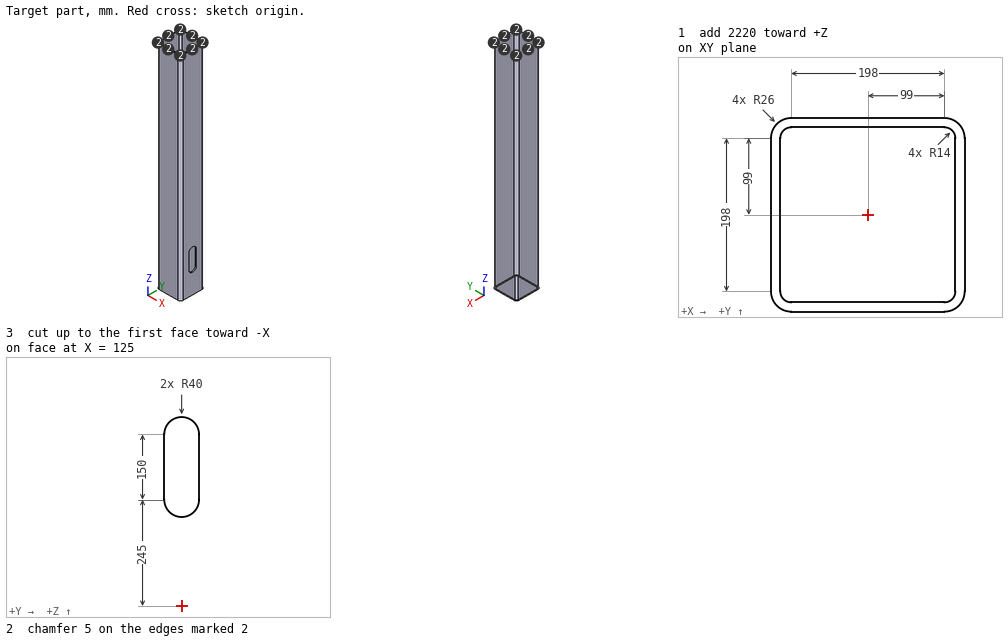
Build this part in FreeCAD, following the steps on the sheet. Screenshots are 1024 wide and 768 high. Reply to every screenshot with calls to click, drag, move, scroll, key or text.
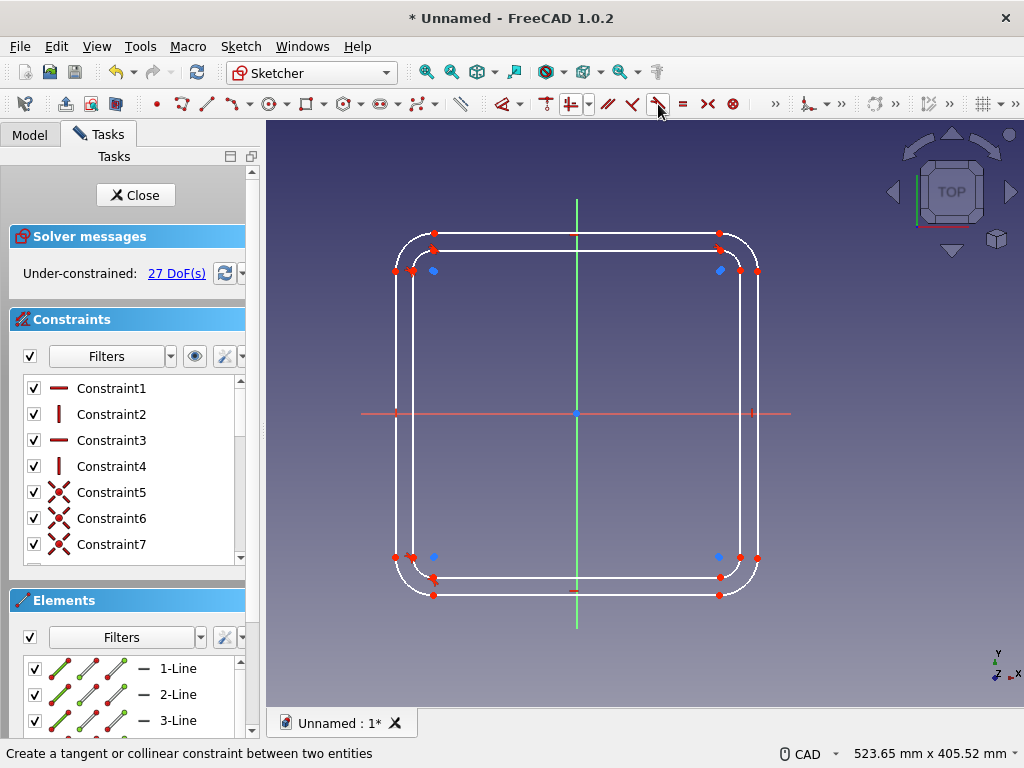
click(520, 595)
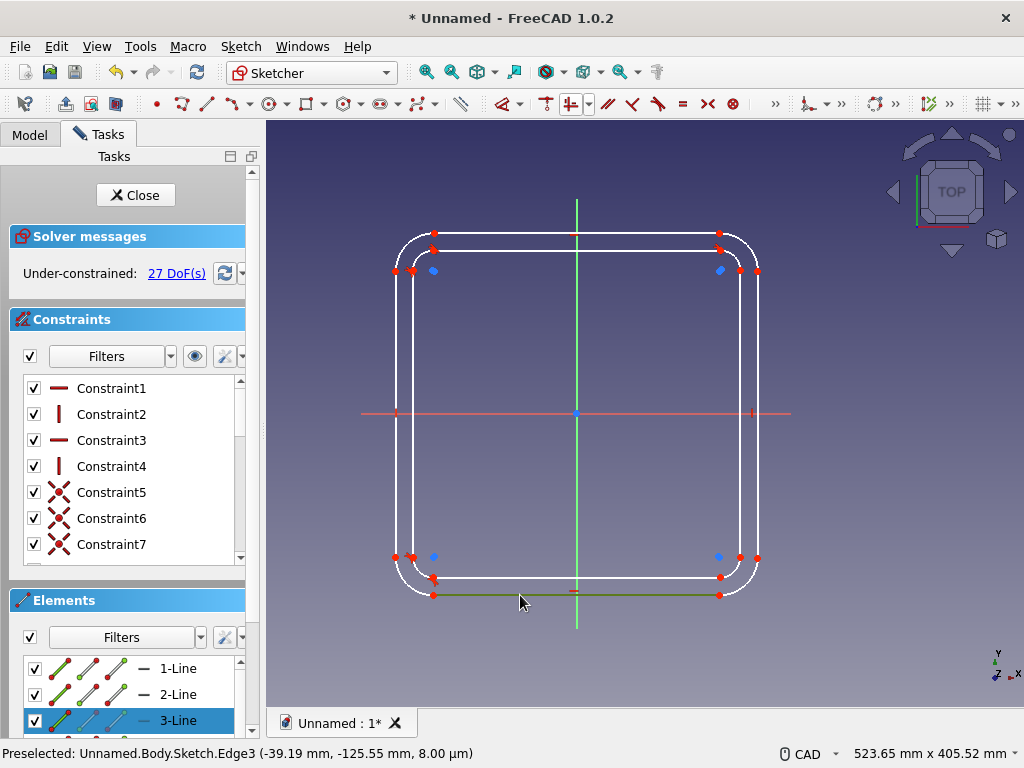
click(737, 591)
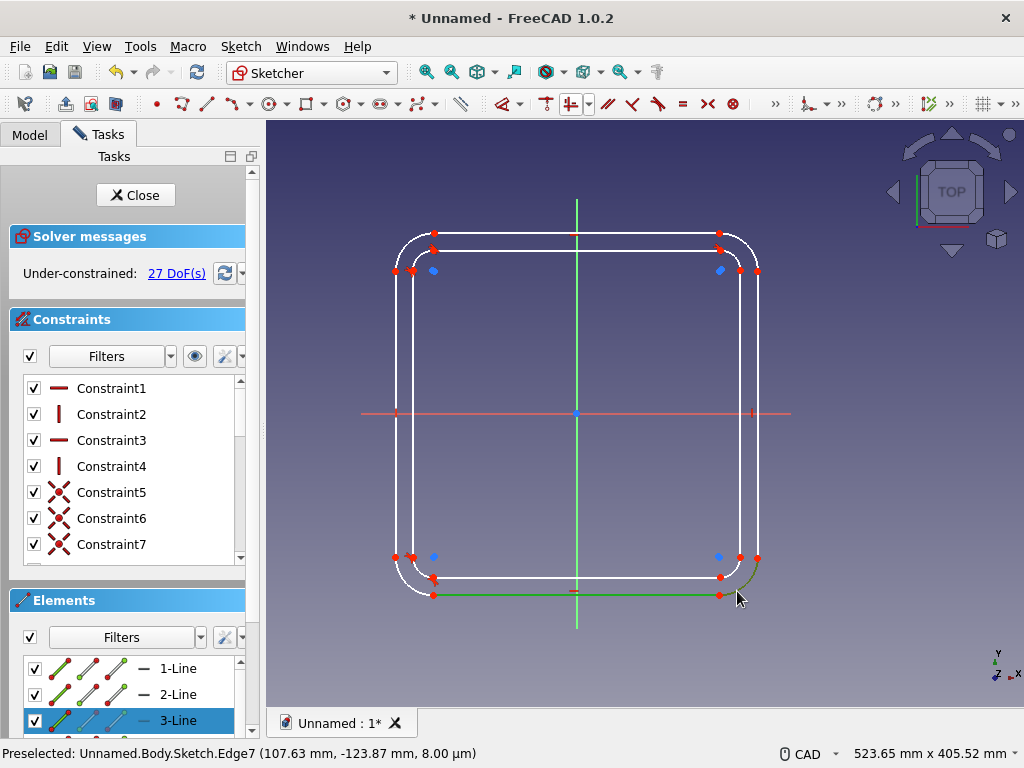
click(658, 104)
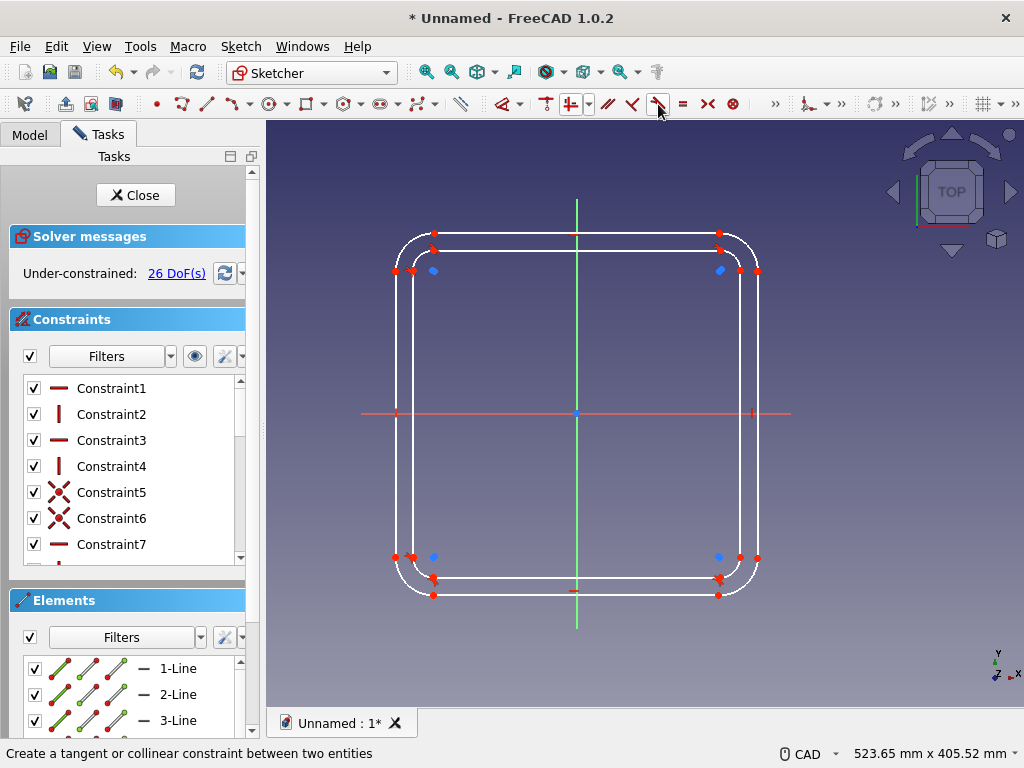
click(758, 472)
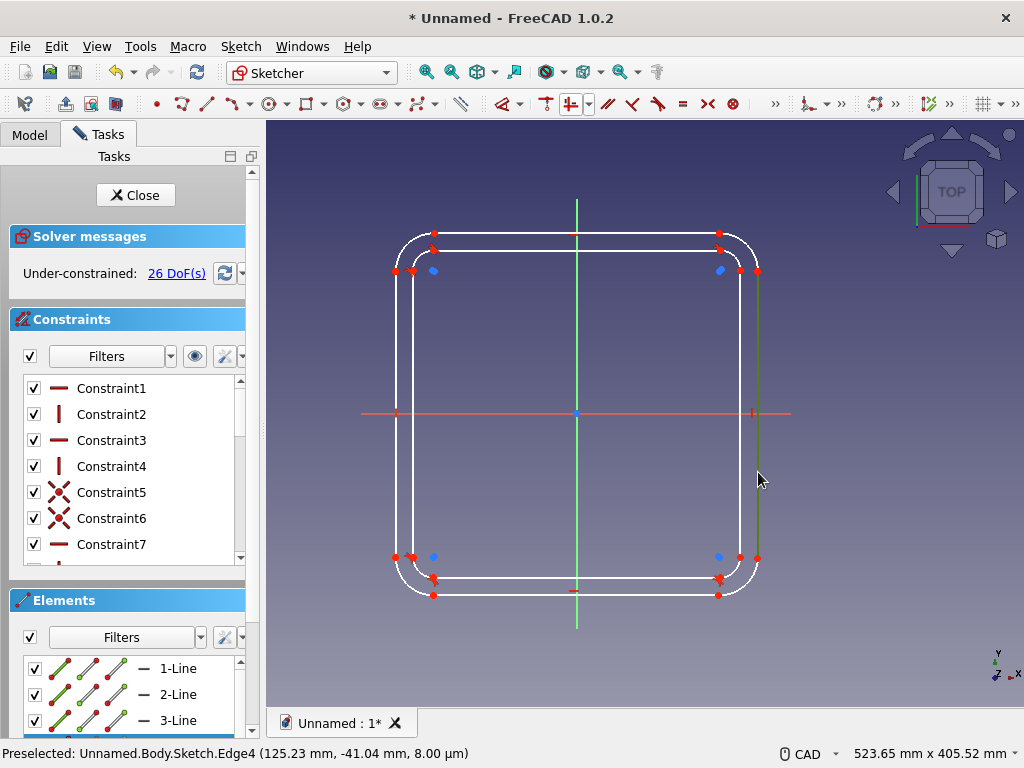
click(736, 591)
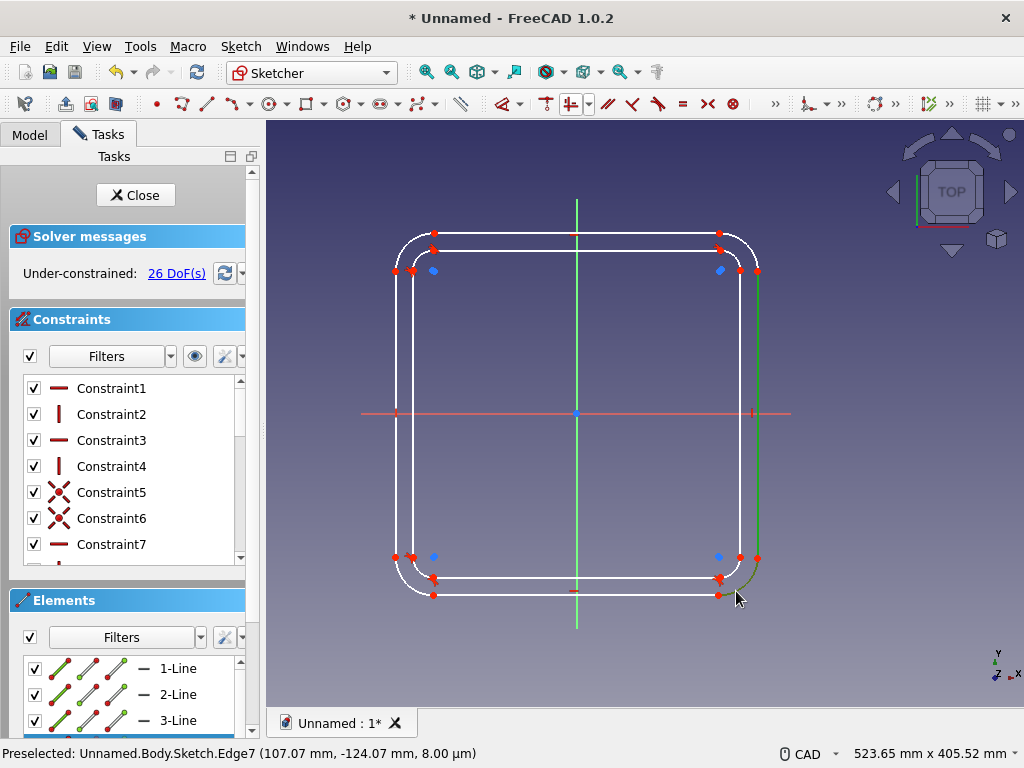
click(658, 104)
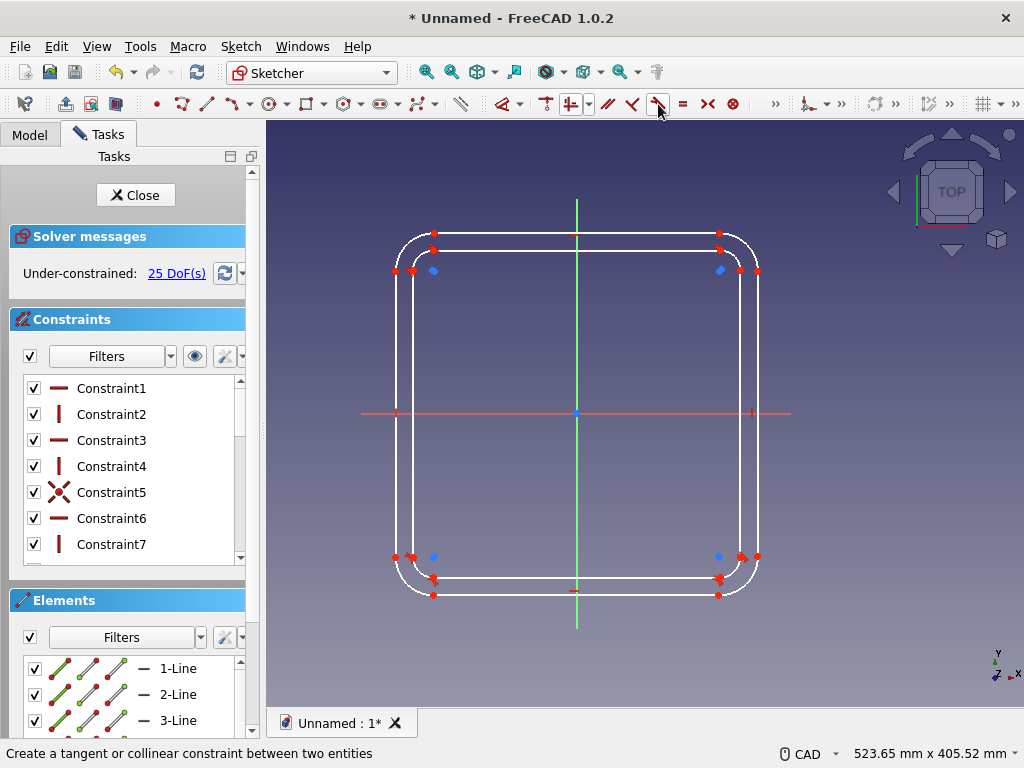
click(758, 471)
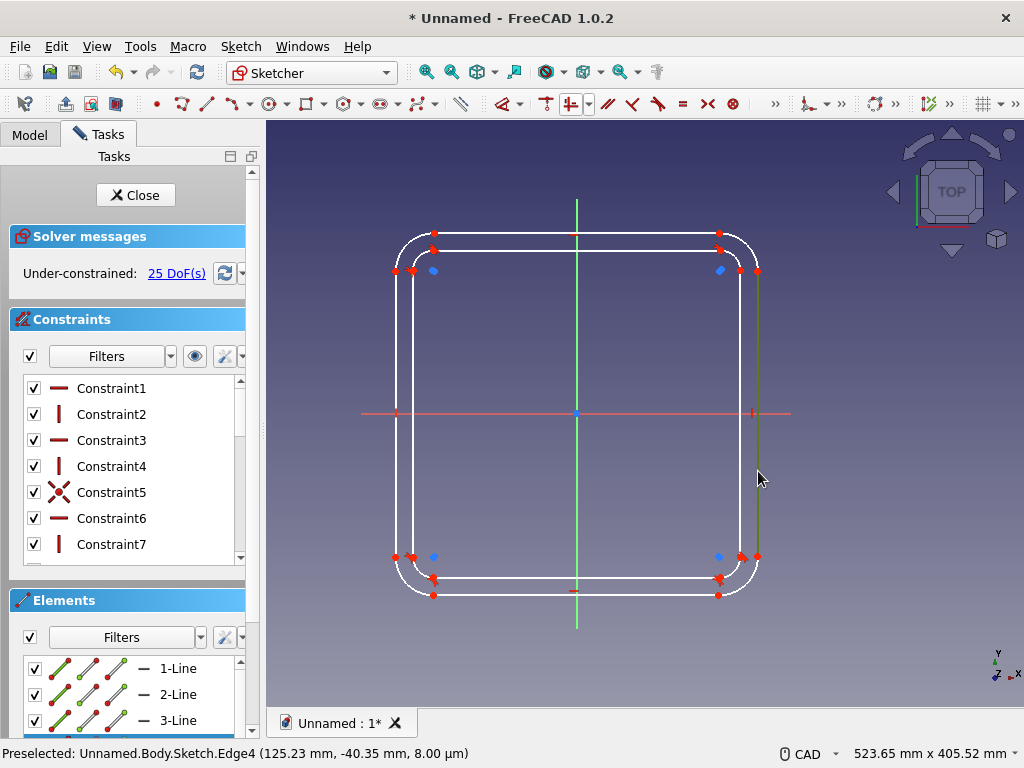
click(754, 254)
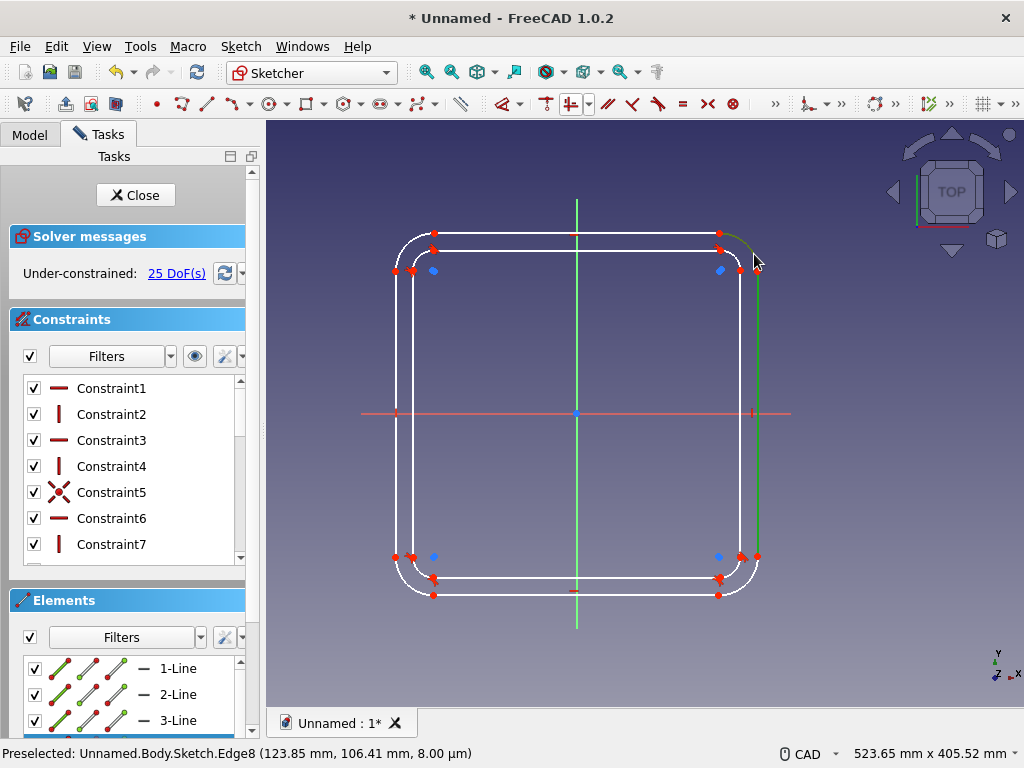
click(658, 104)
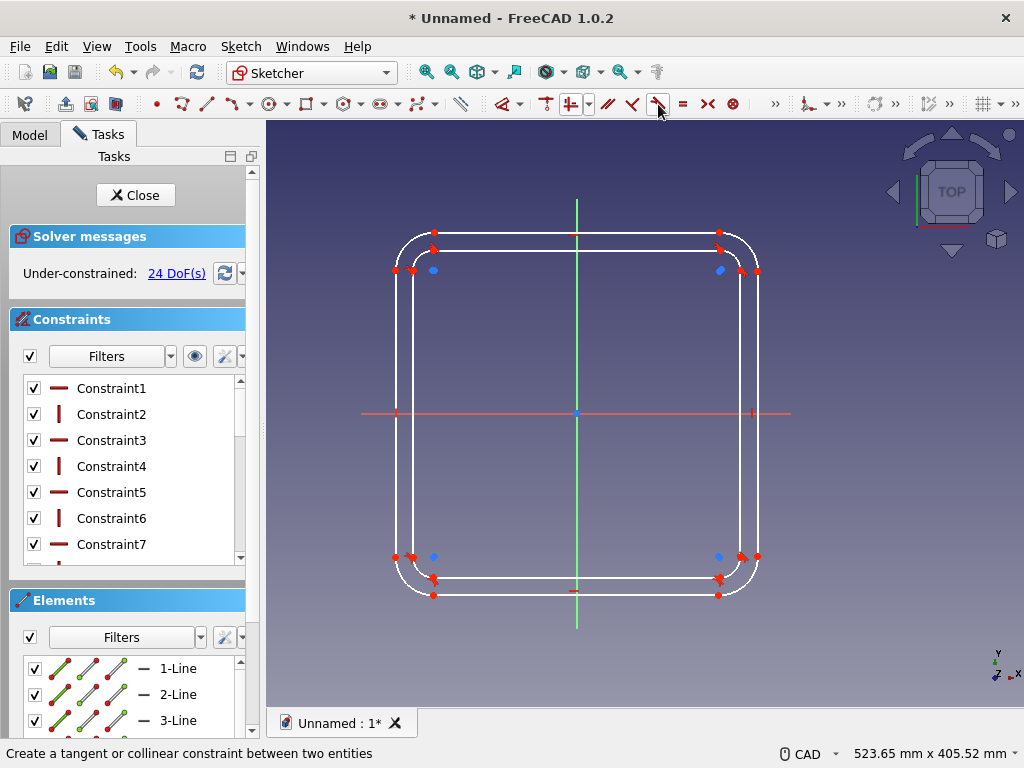
click(519, 251)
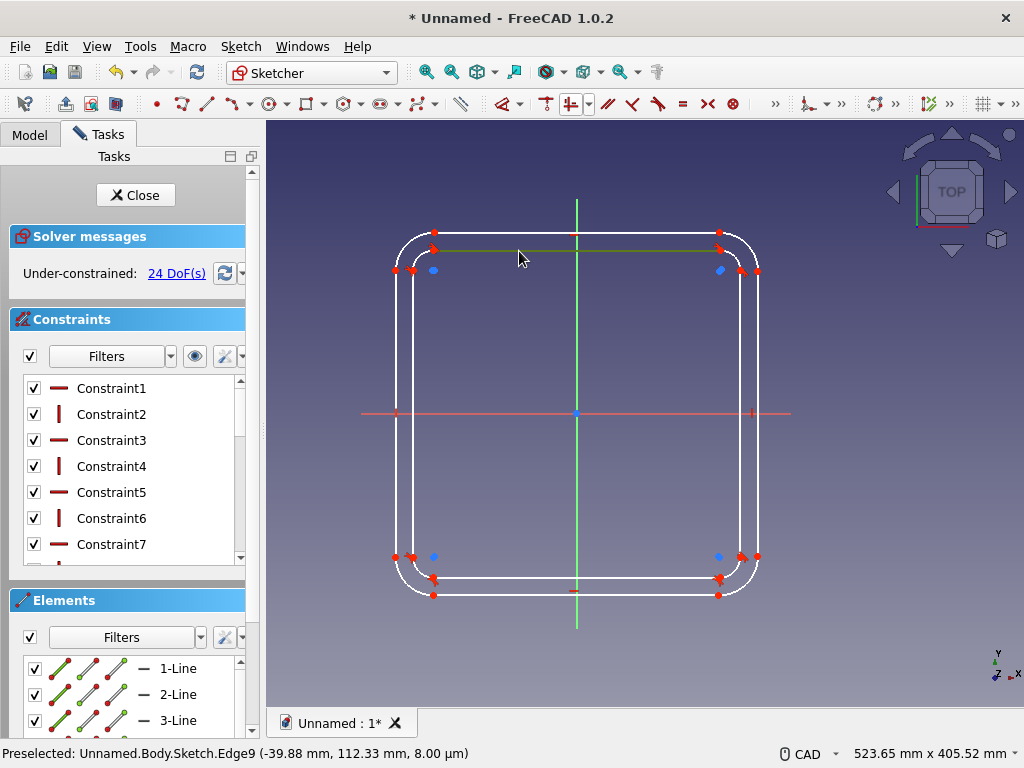
scroll(738, 262, up, 2)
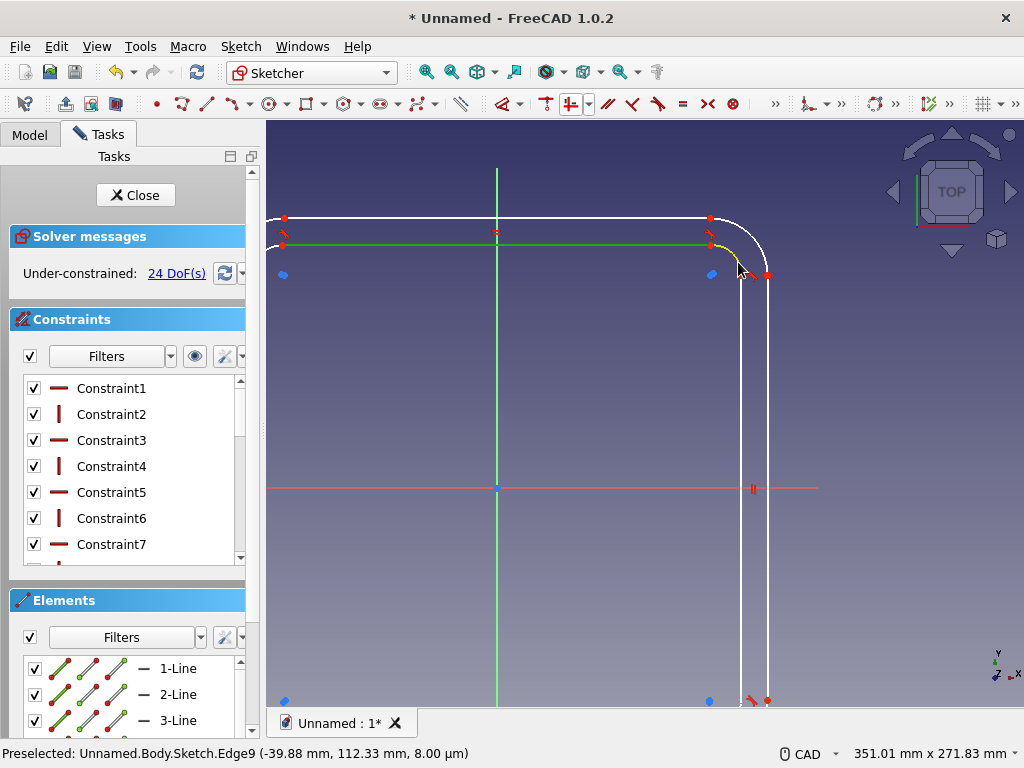
click(738, 261)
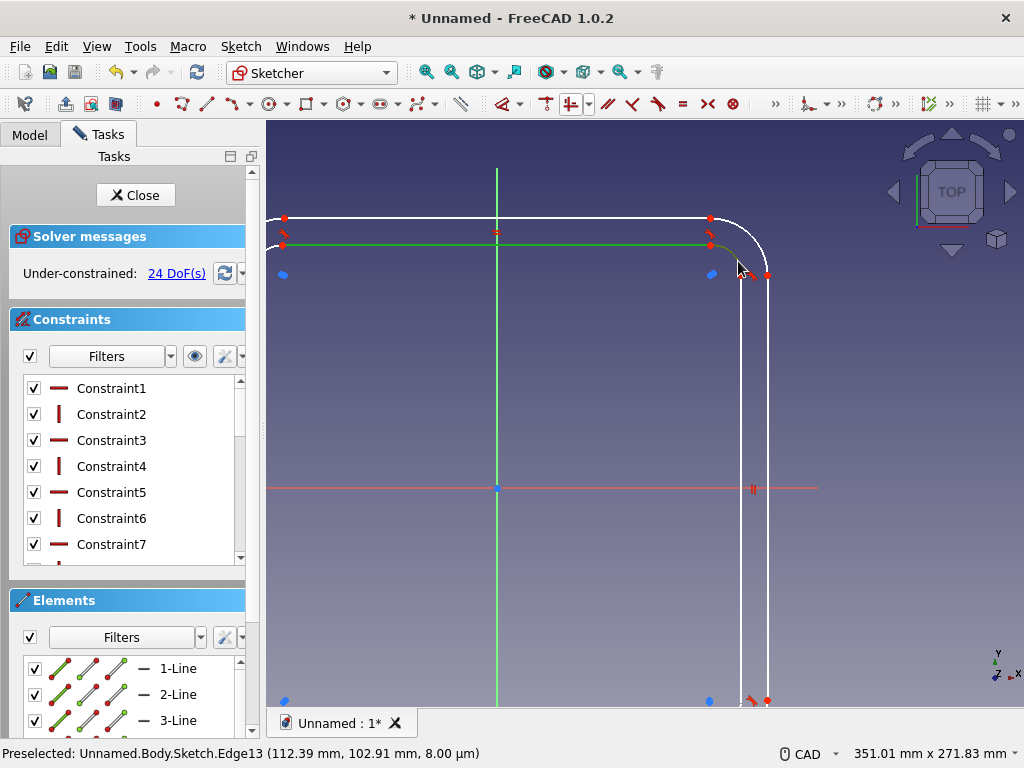
click(658, 104)